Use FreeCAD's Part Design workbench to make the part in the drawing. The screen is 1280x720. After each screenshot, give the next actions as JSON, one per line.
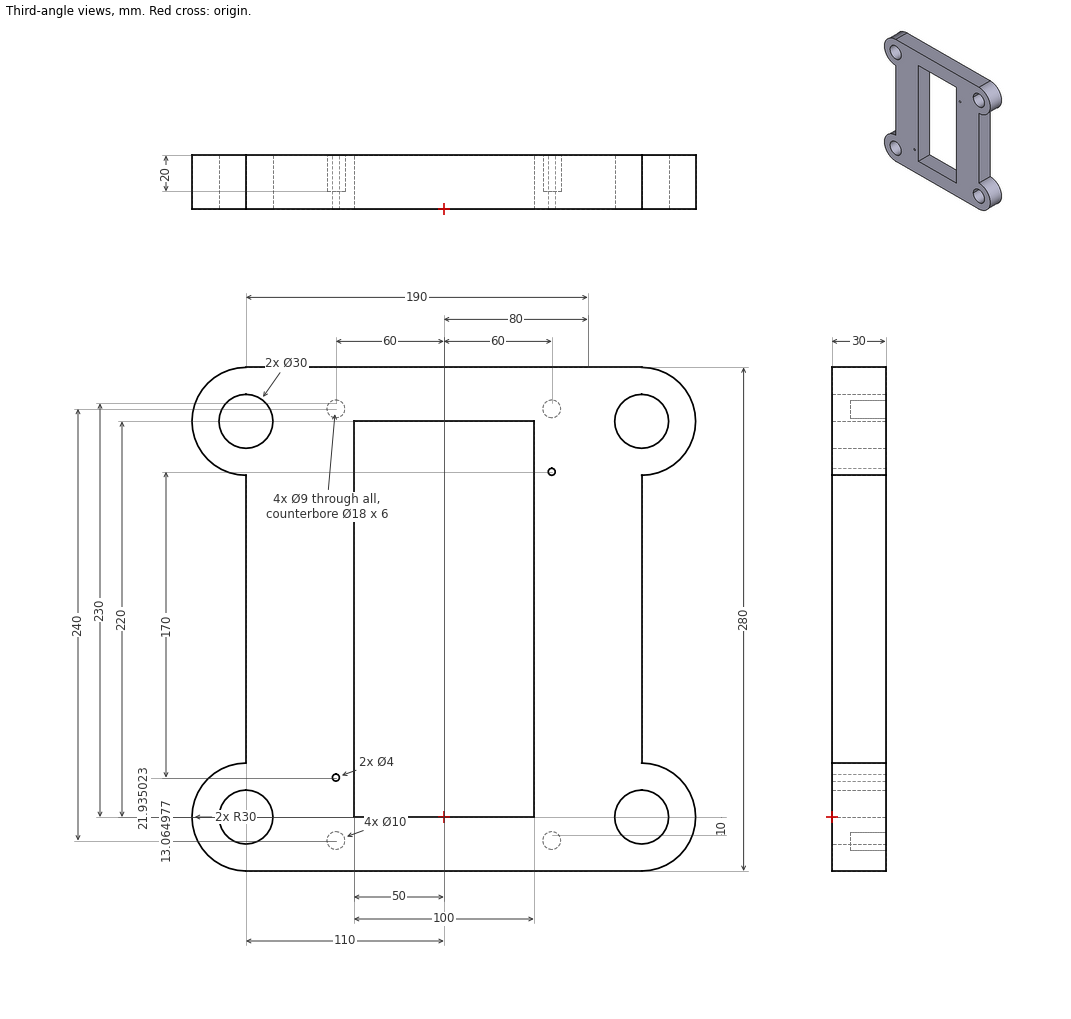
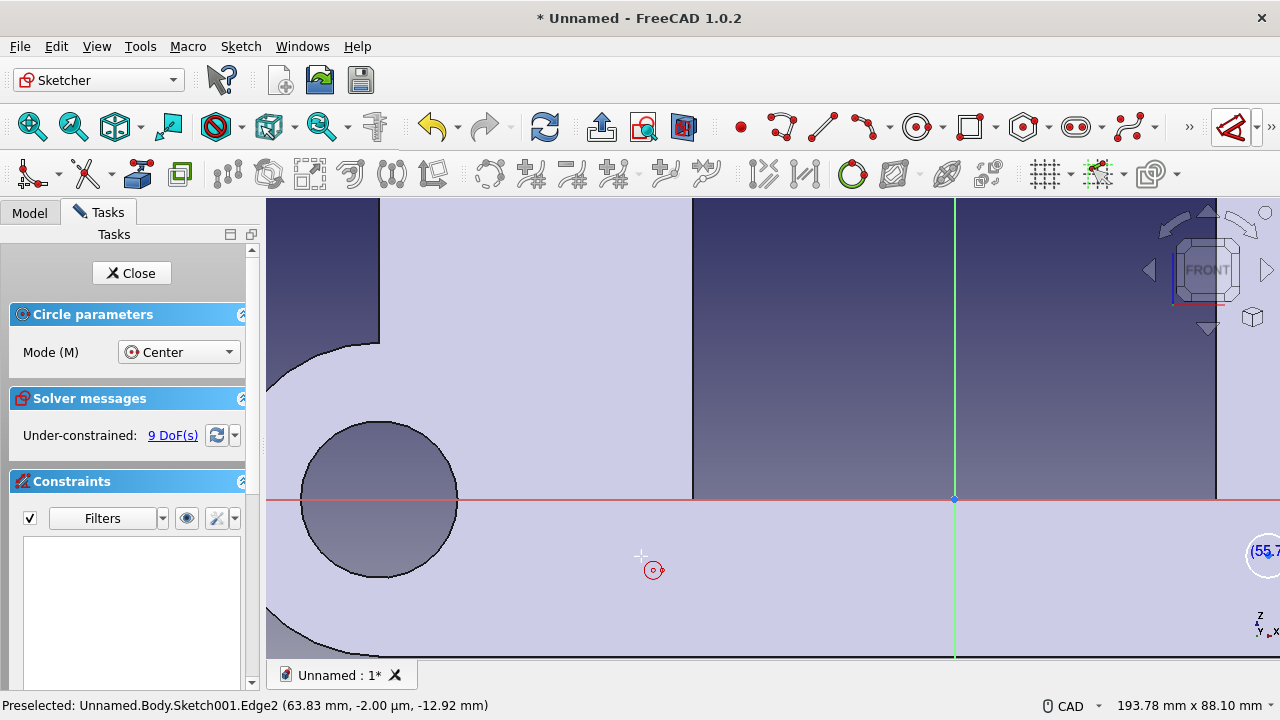
{"action": "scroll", "coordinate": [641, 556], "scroll_direction": "down", "scroll_amount": 8}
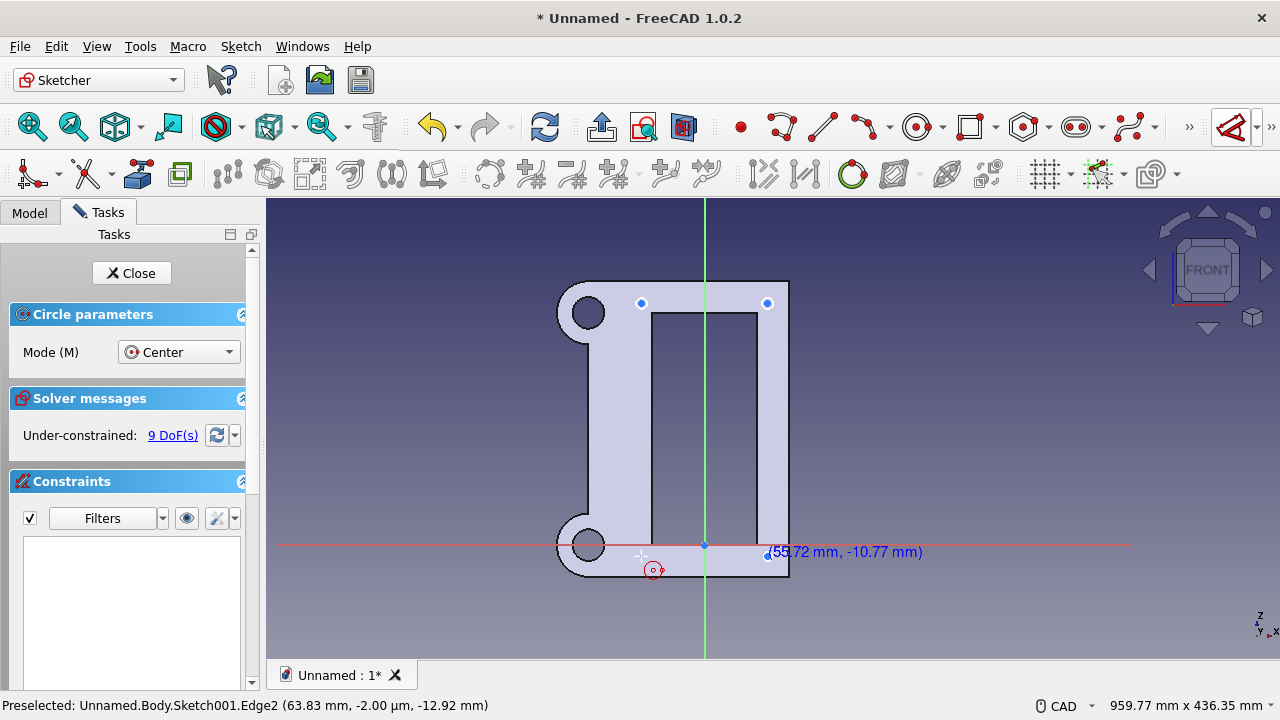
{"action": "scroll", "coordinate": [641, 556], "scroll_direction": "up", "scroll_amount": 3}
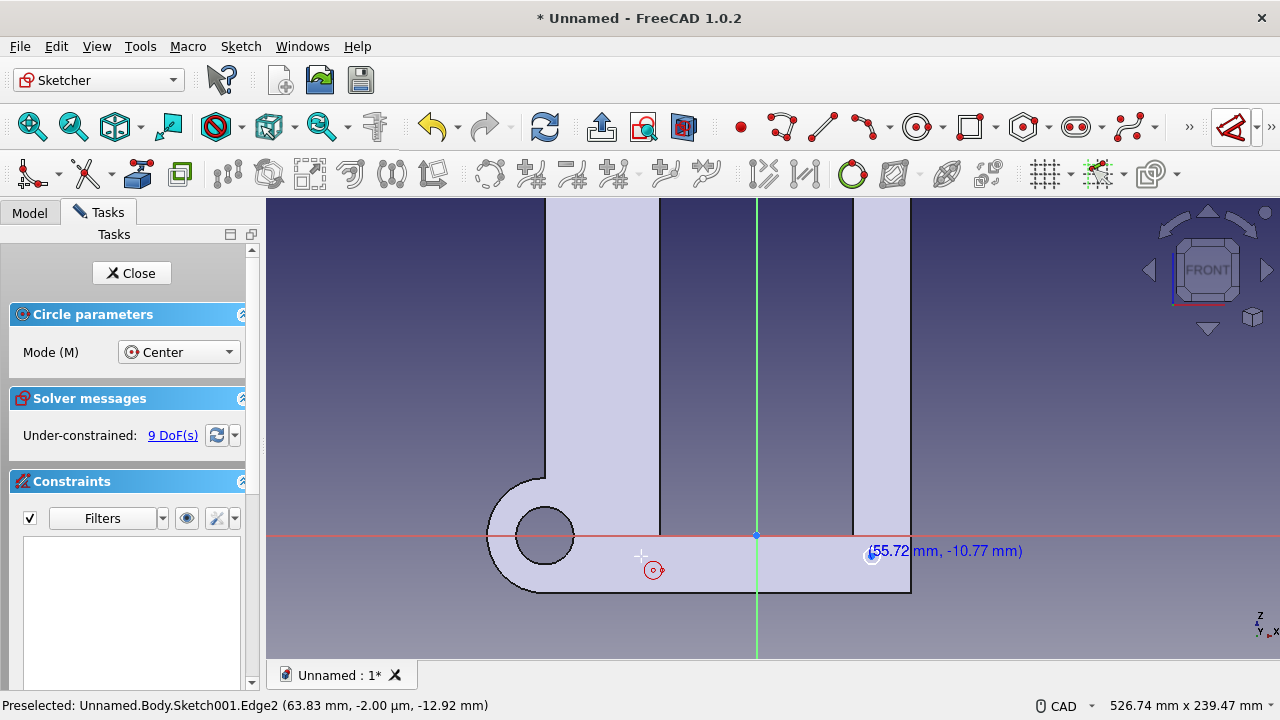
{"action": "left_click", "coordinate": [641, 555]}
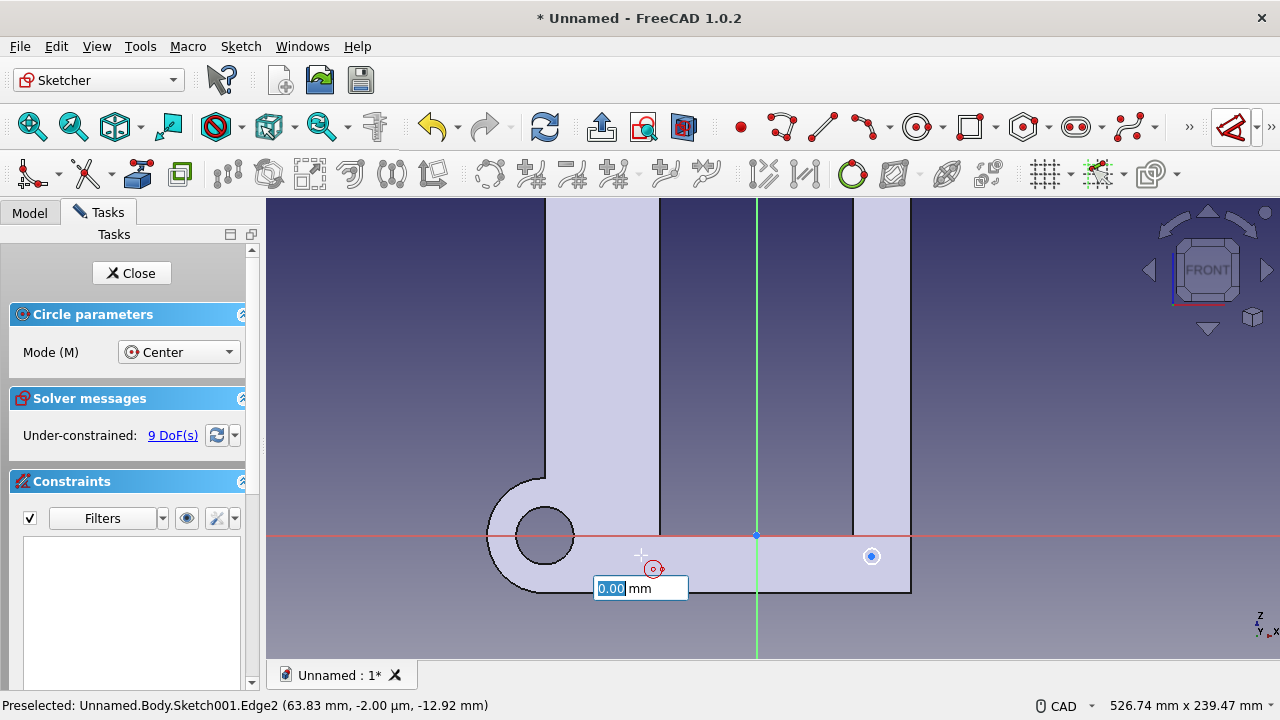
{"action": "scroll", "coordinate": [647, 561], "scroll_direction": "up", "scroll_amount": 4}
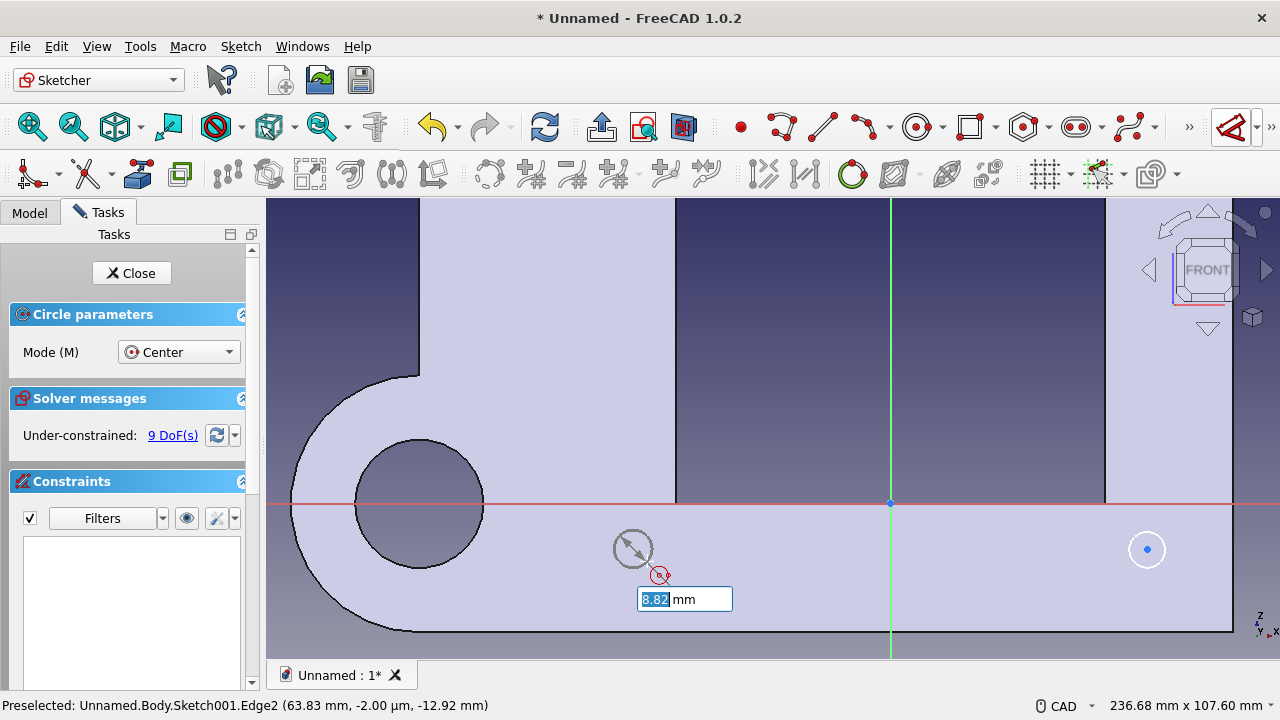
{"action": "left_click", "coordinate": [647, 560]}
{"action": "key", "text": "Escape"}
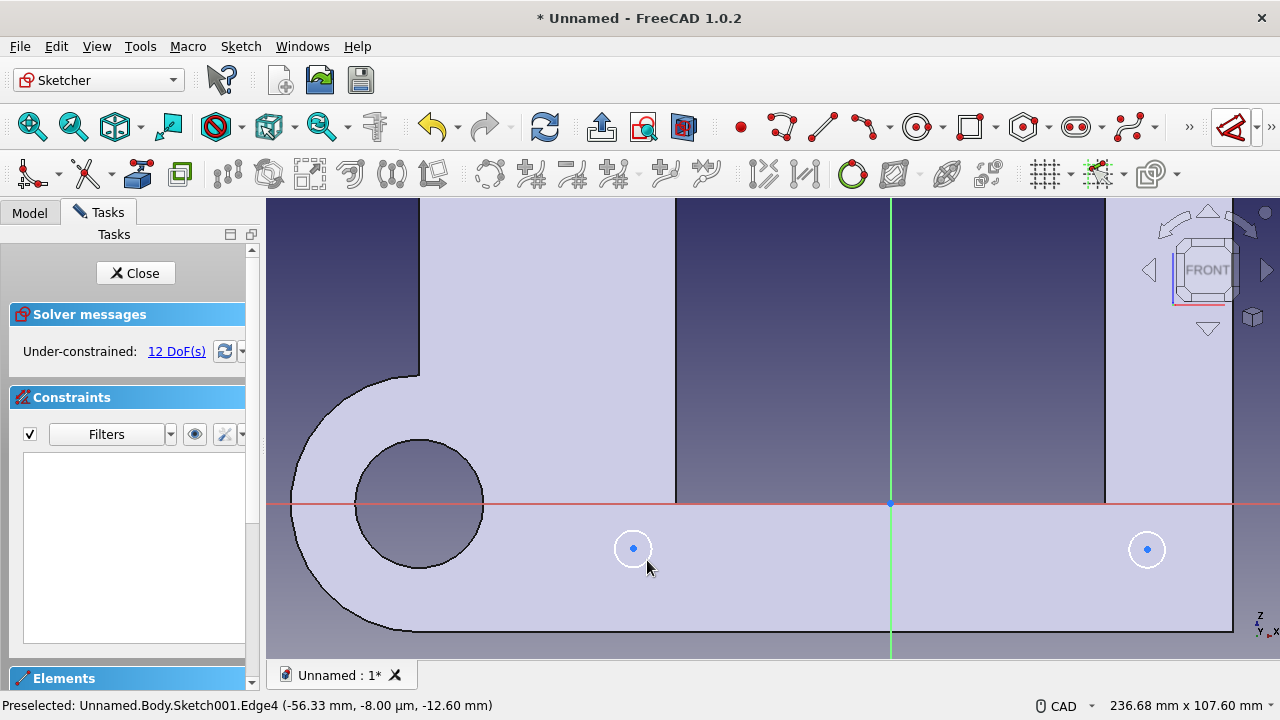
{"action": "scroll", "coordinate": [644, 558], "scroll_direction": "down", "scroll_amount": 7}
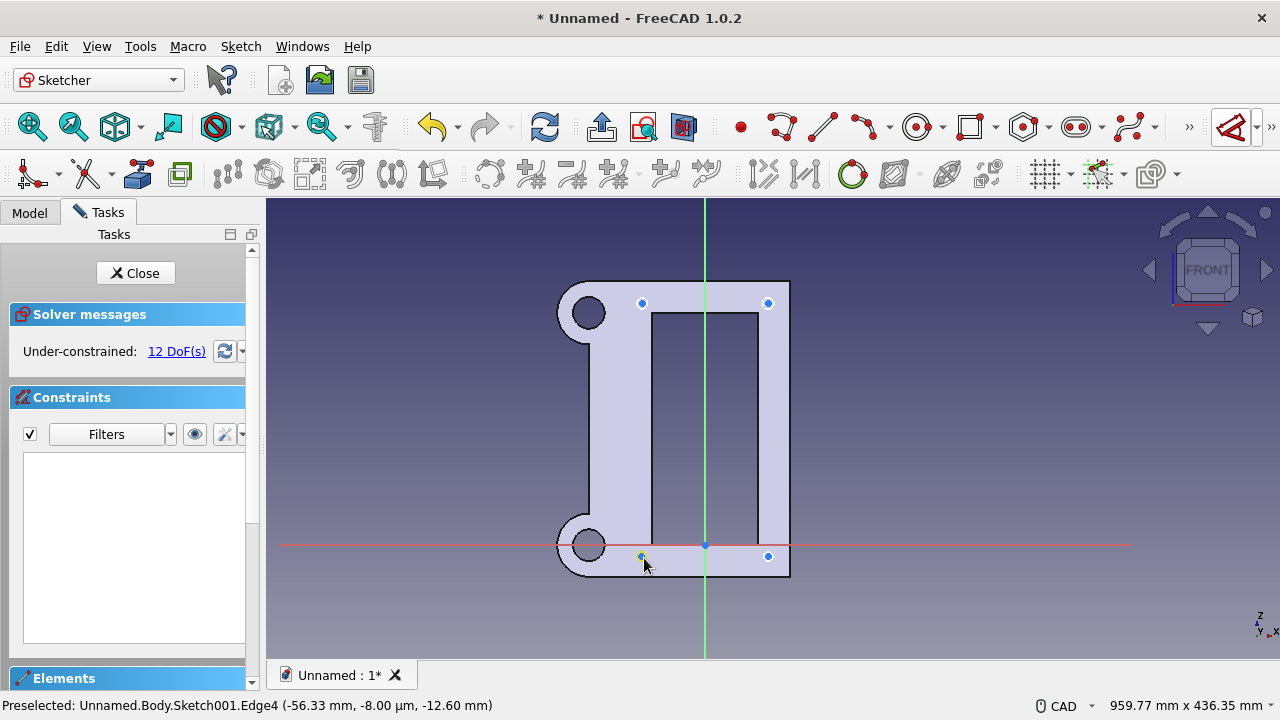
{"action": "scroll", "coordinate": [646, 300], "scroll_direction": "up", "scroll_amount": 5}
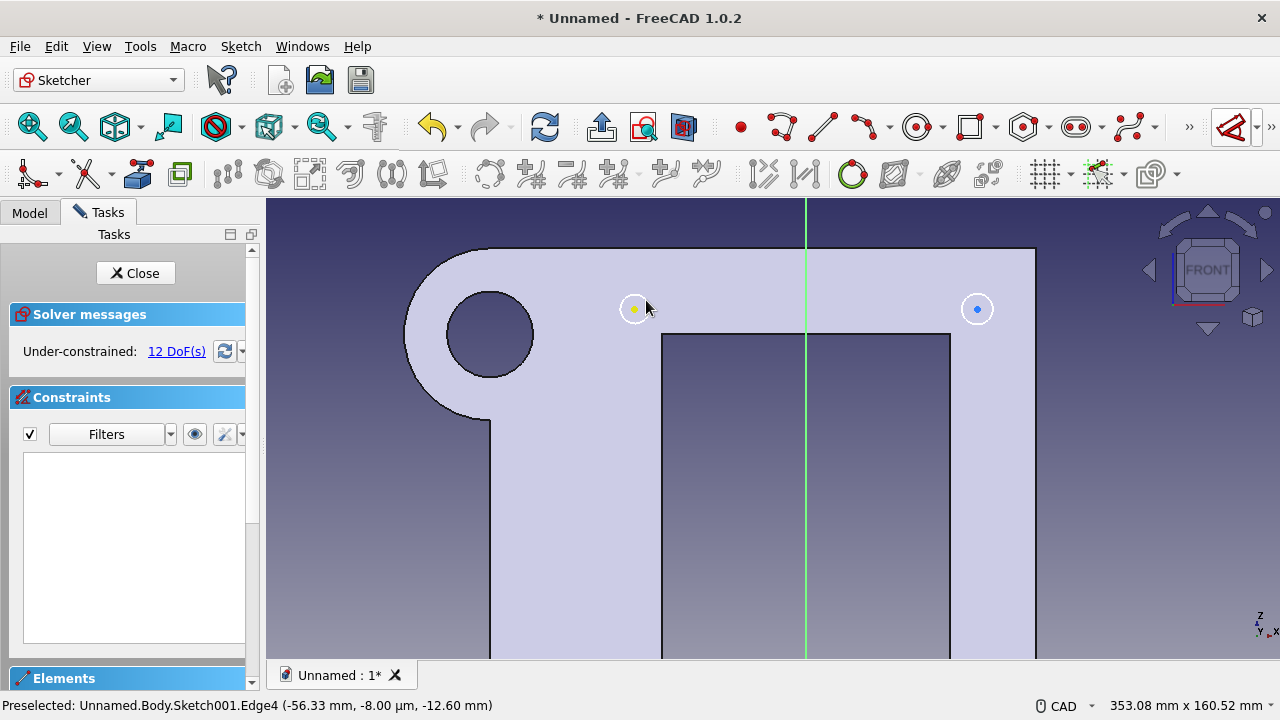
{"action": "left_click", "coordinate": [645, 299]}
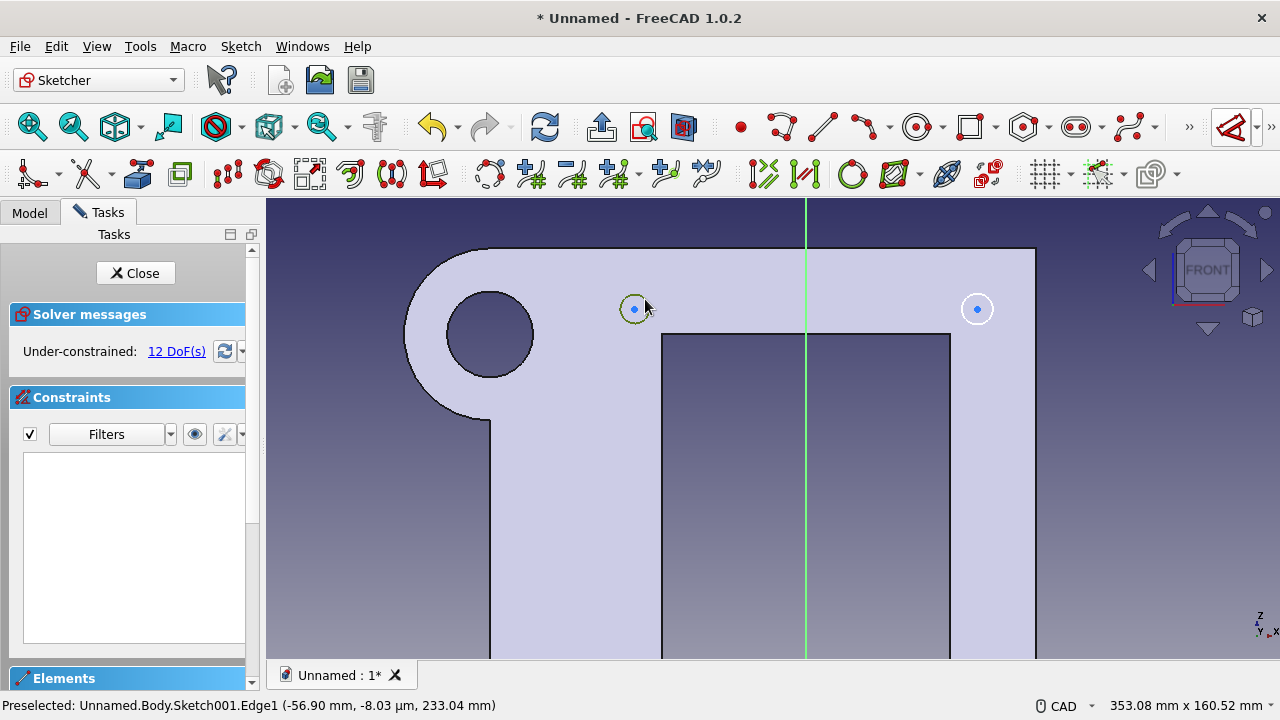
{"action": "left_click", "coordinate": [988, 298]}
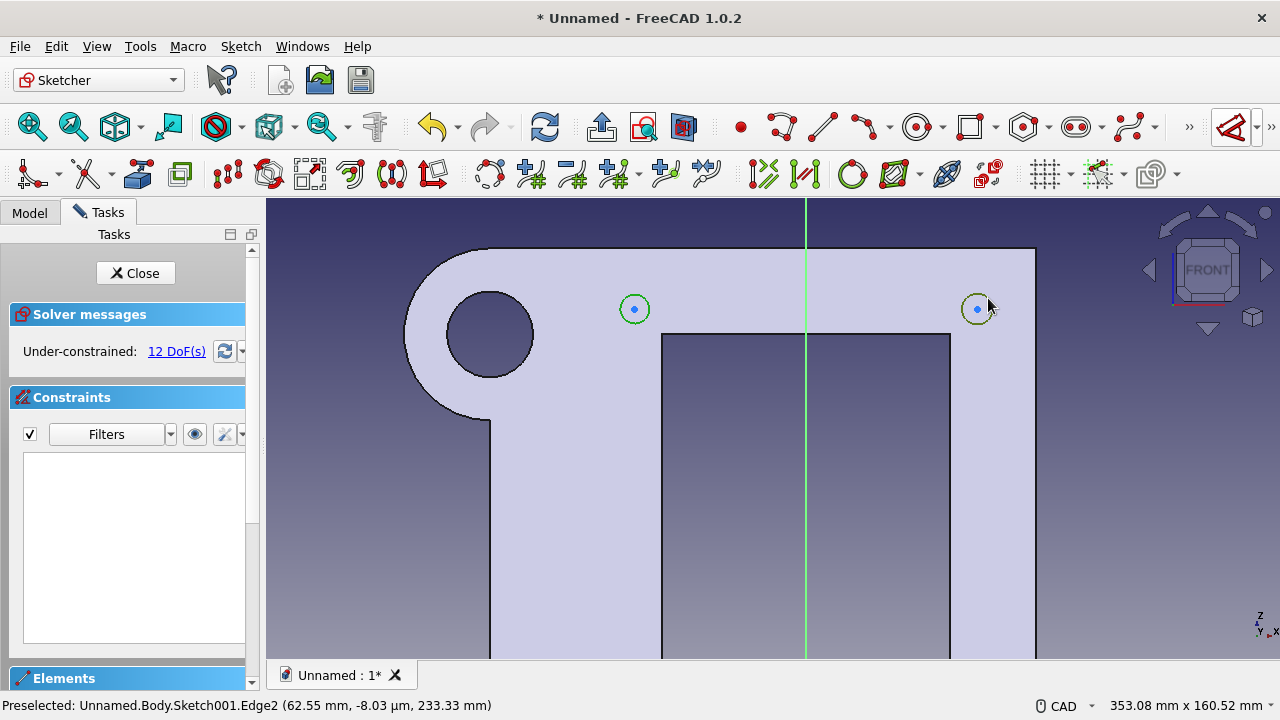
{"action": "scroll", "coordinate": [645, 299], "scroll_direction": "down", "scroll_amount": 5}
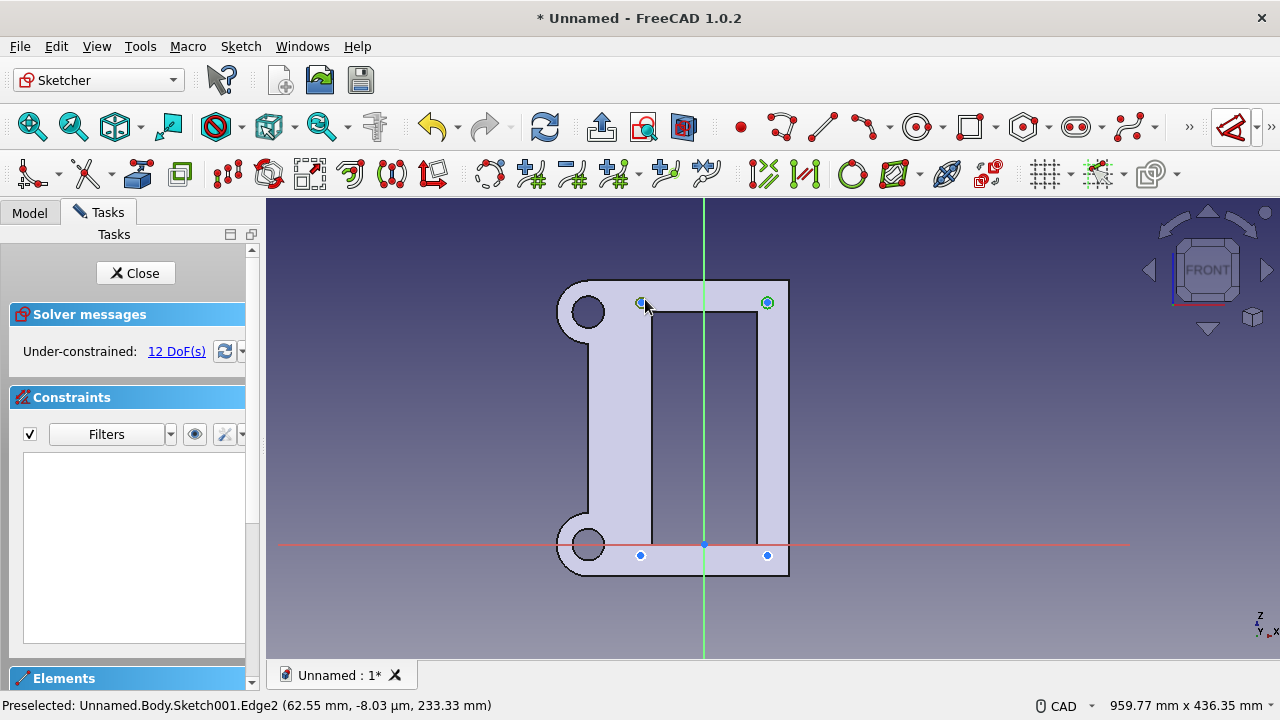
{"action": "scroll", "coordinate": [771, 553], "scroll_direction": "up", "scroll_amount": 6}